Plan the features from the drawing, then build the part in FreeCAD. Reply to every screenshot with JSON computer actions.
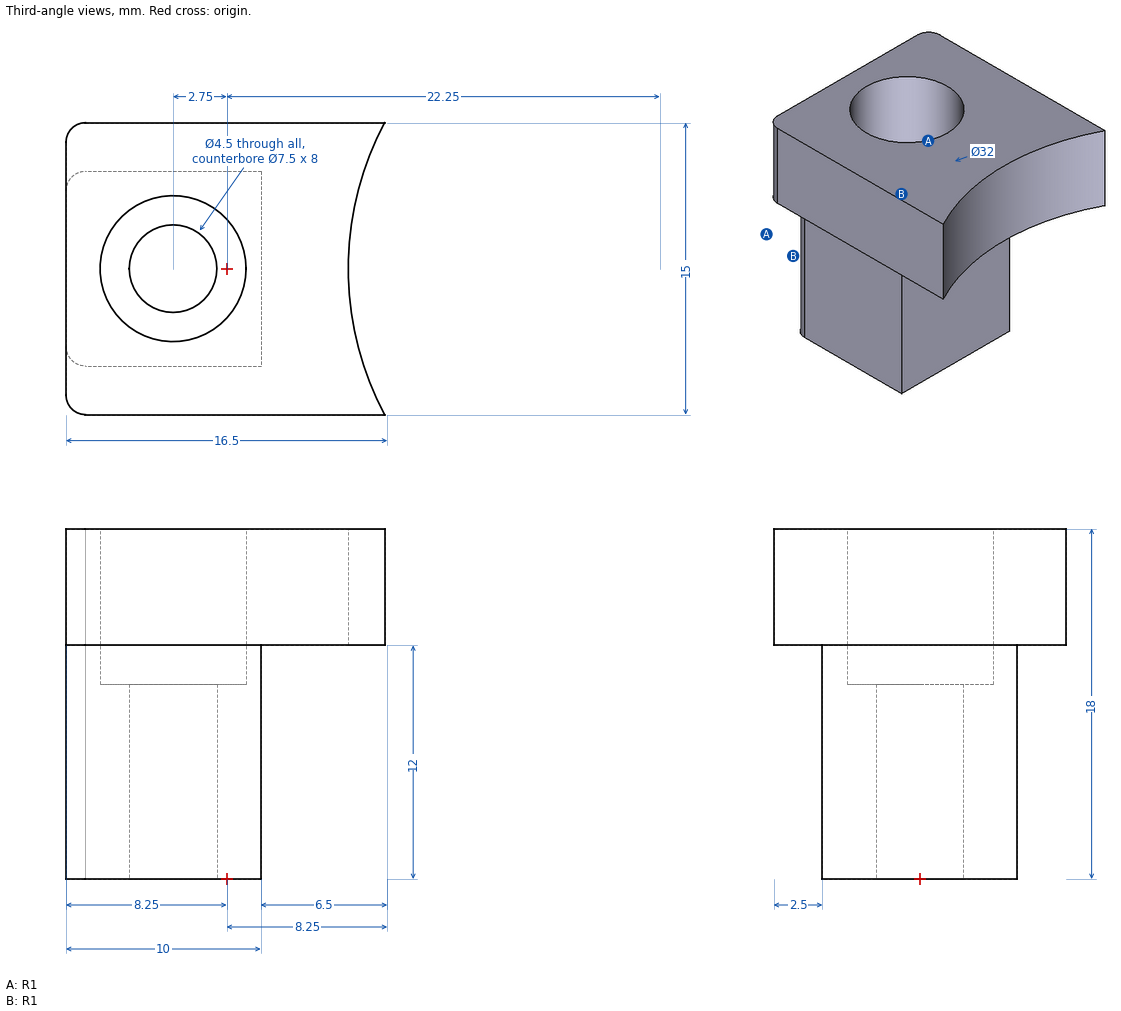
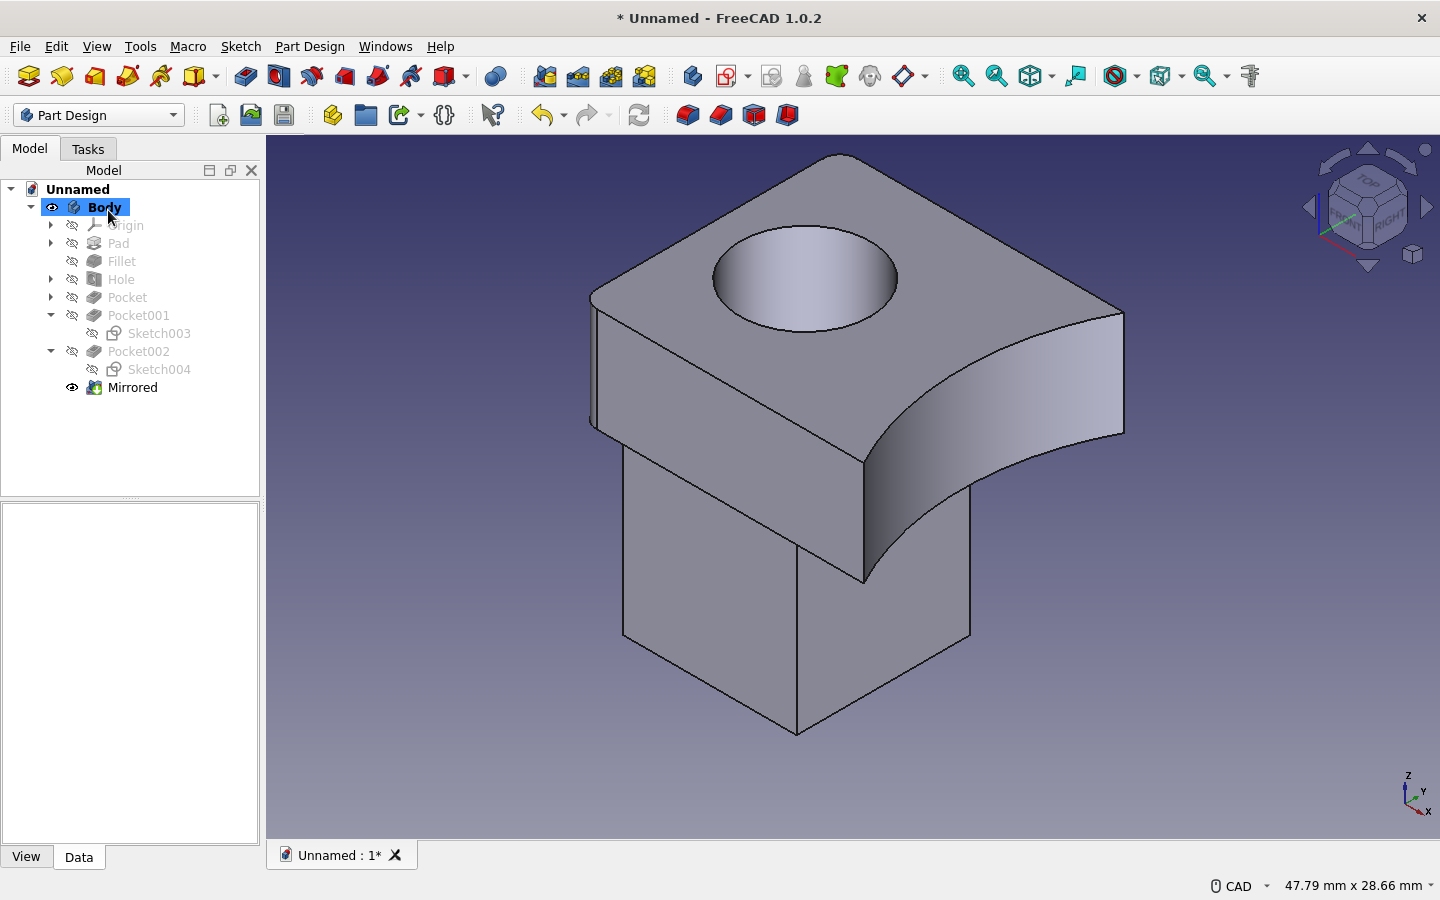
{"action": "key", "text": "1"}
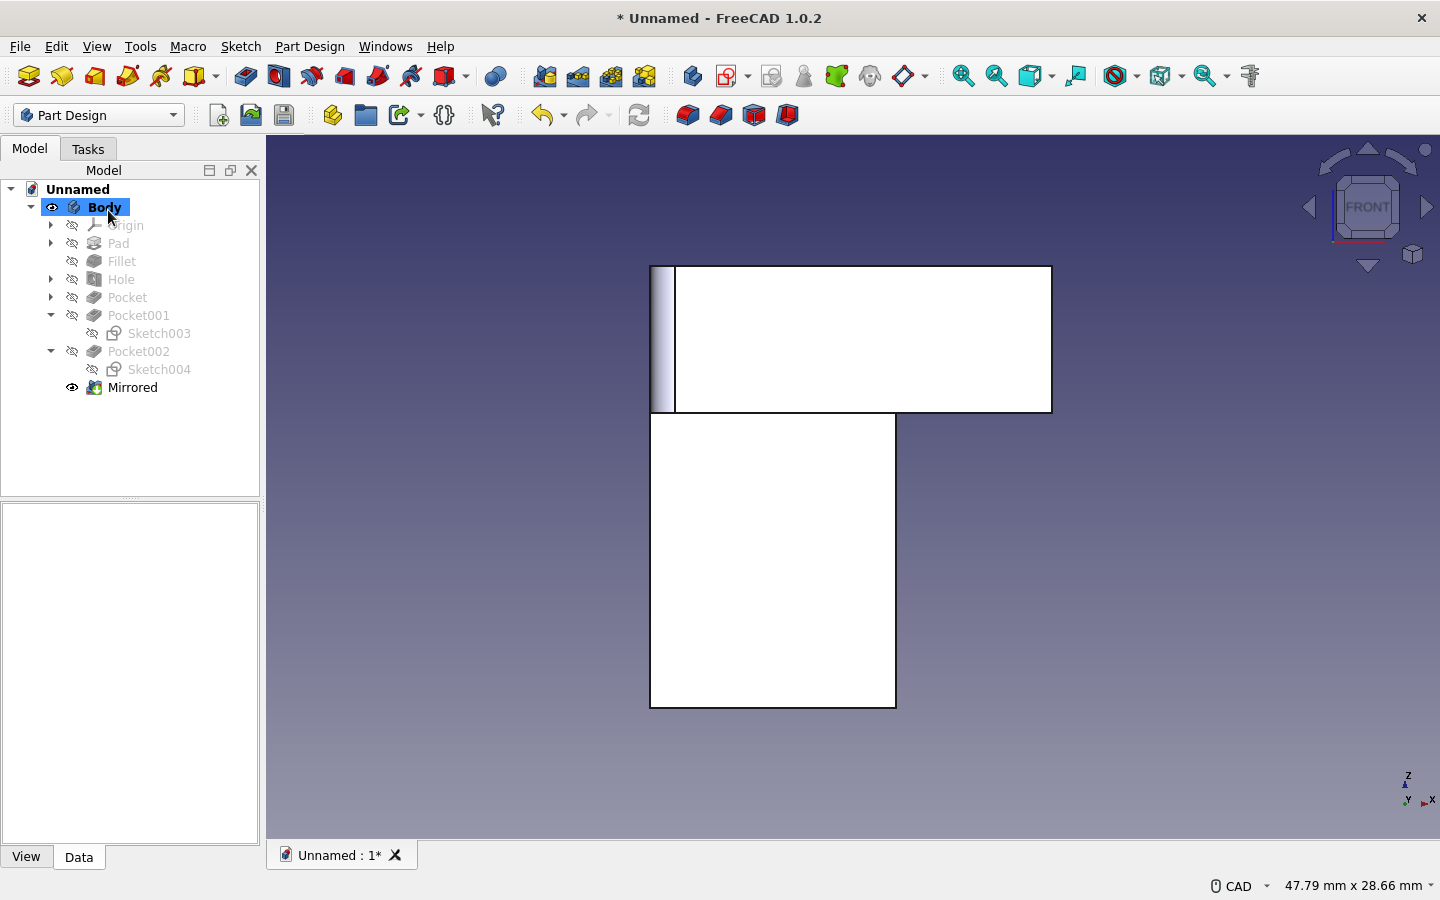
{"action": "left_click", "coordinate": [650, 560]}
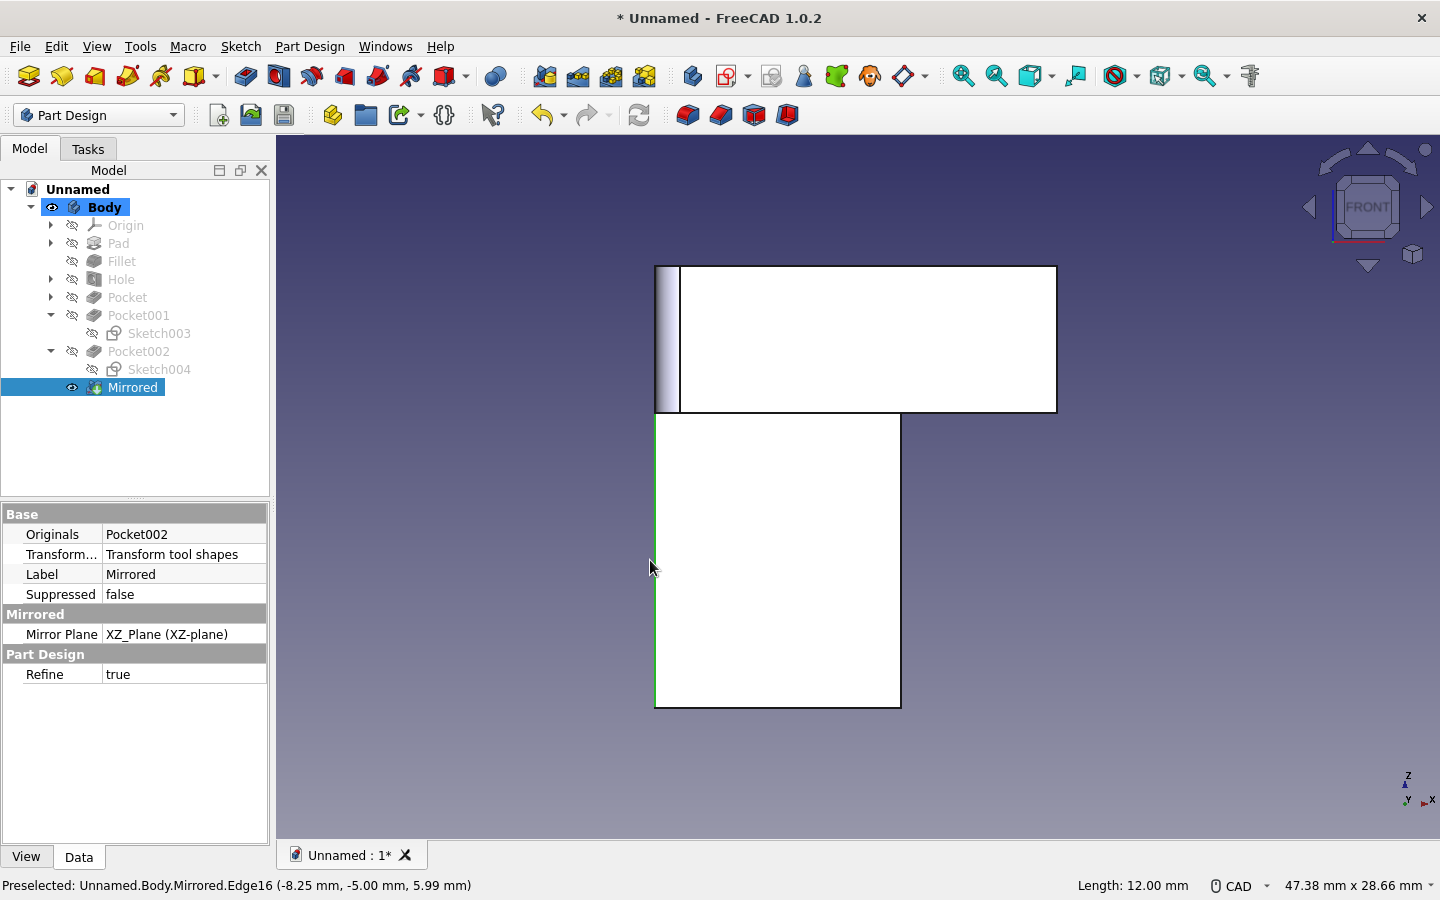
{"action": "key", "text": "3"}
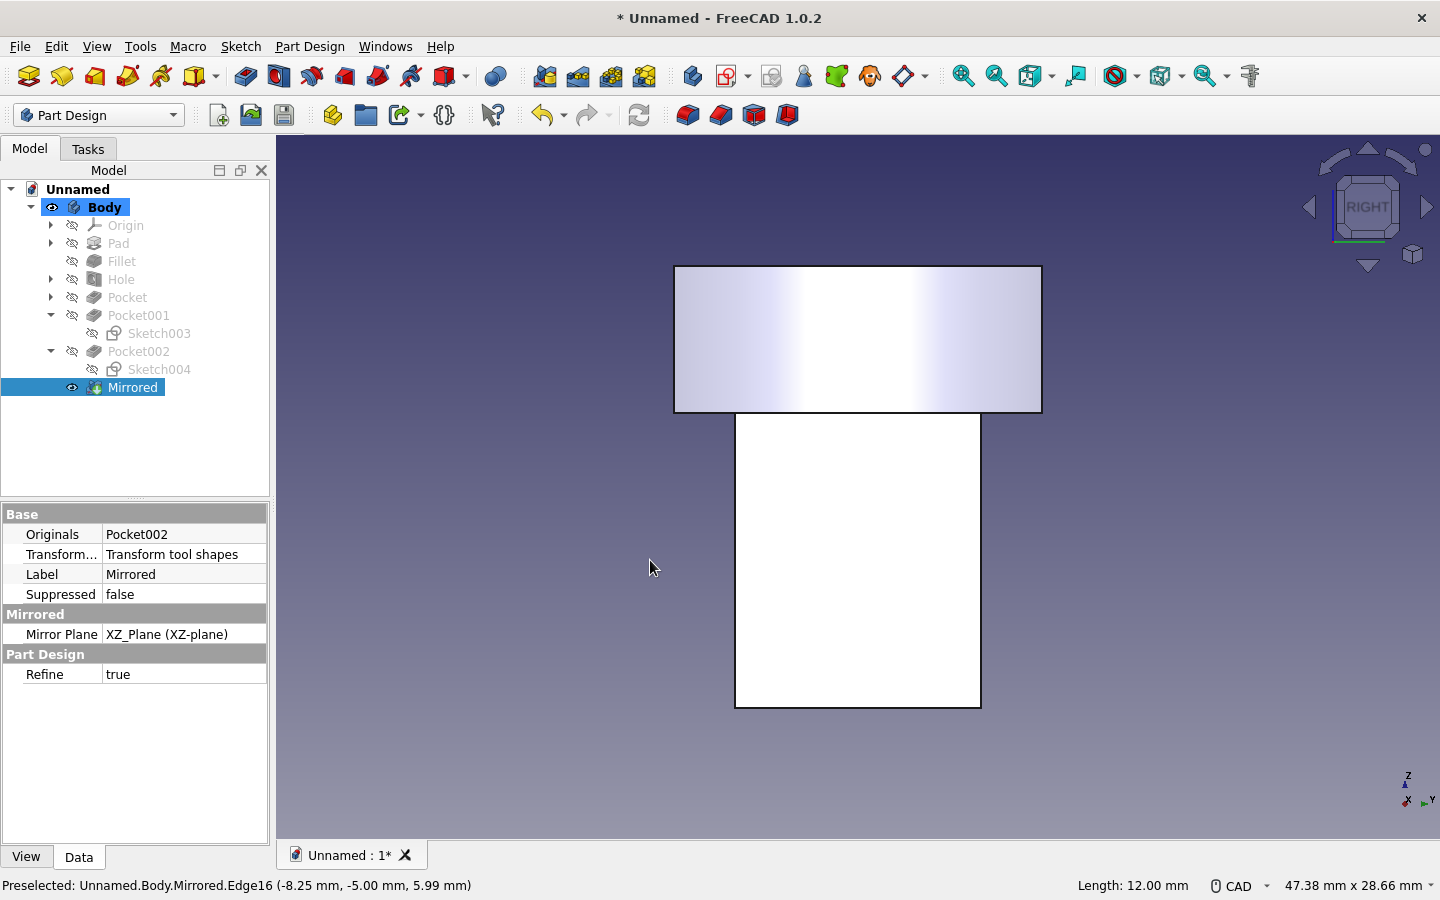
{"action": "key", "text": "5"}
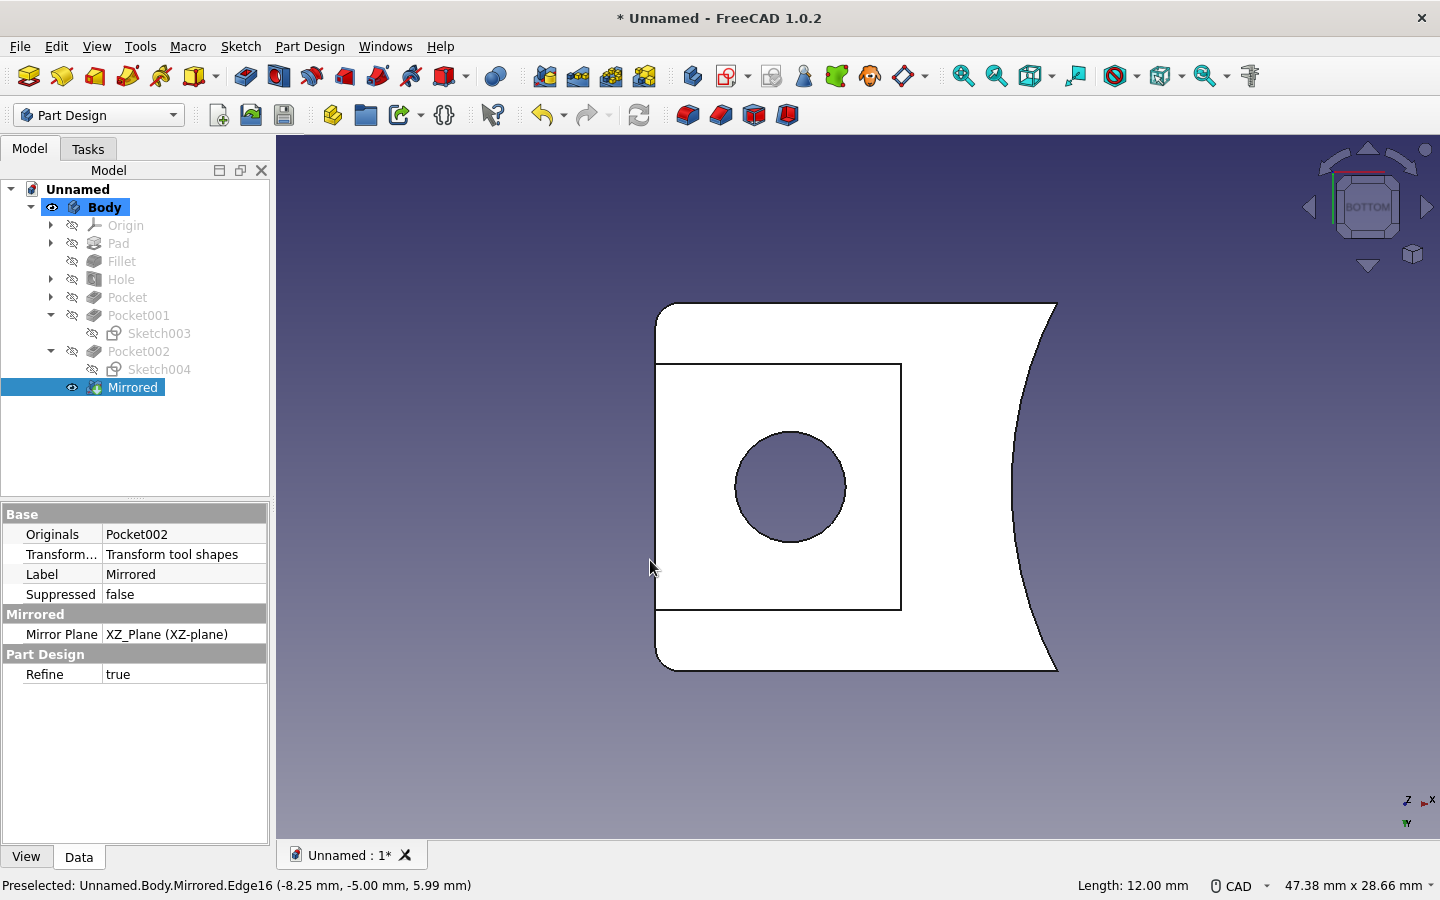
{"action": "key", "text": "4"}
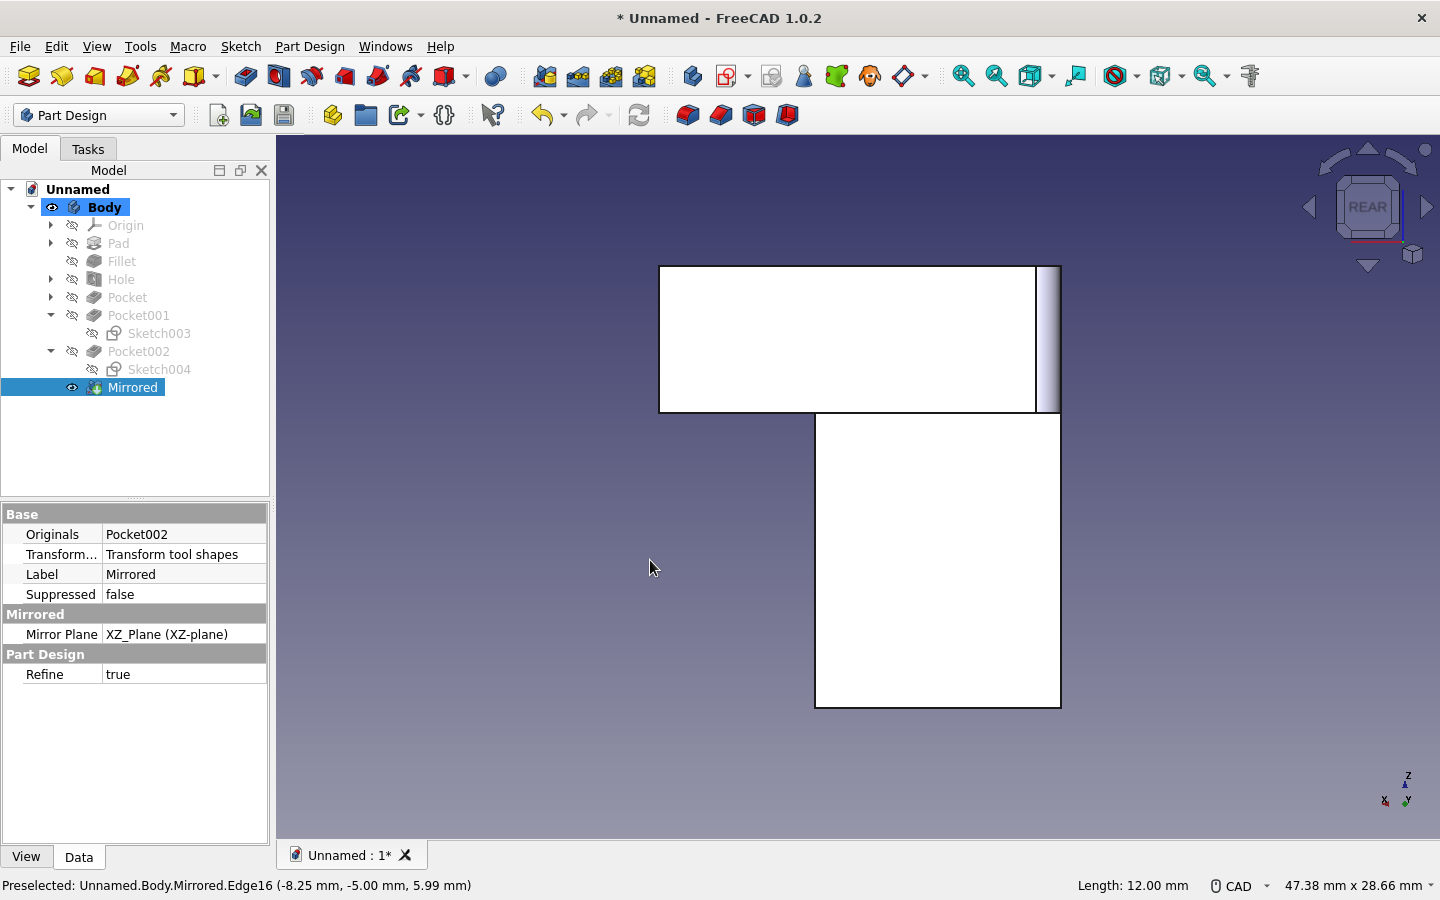
{"action": "left_click", "coordinate": [1061, 560], "text": "ctrl"}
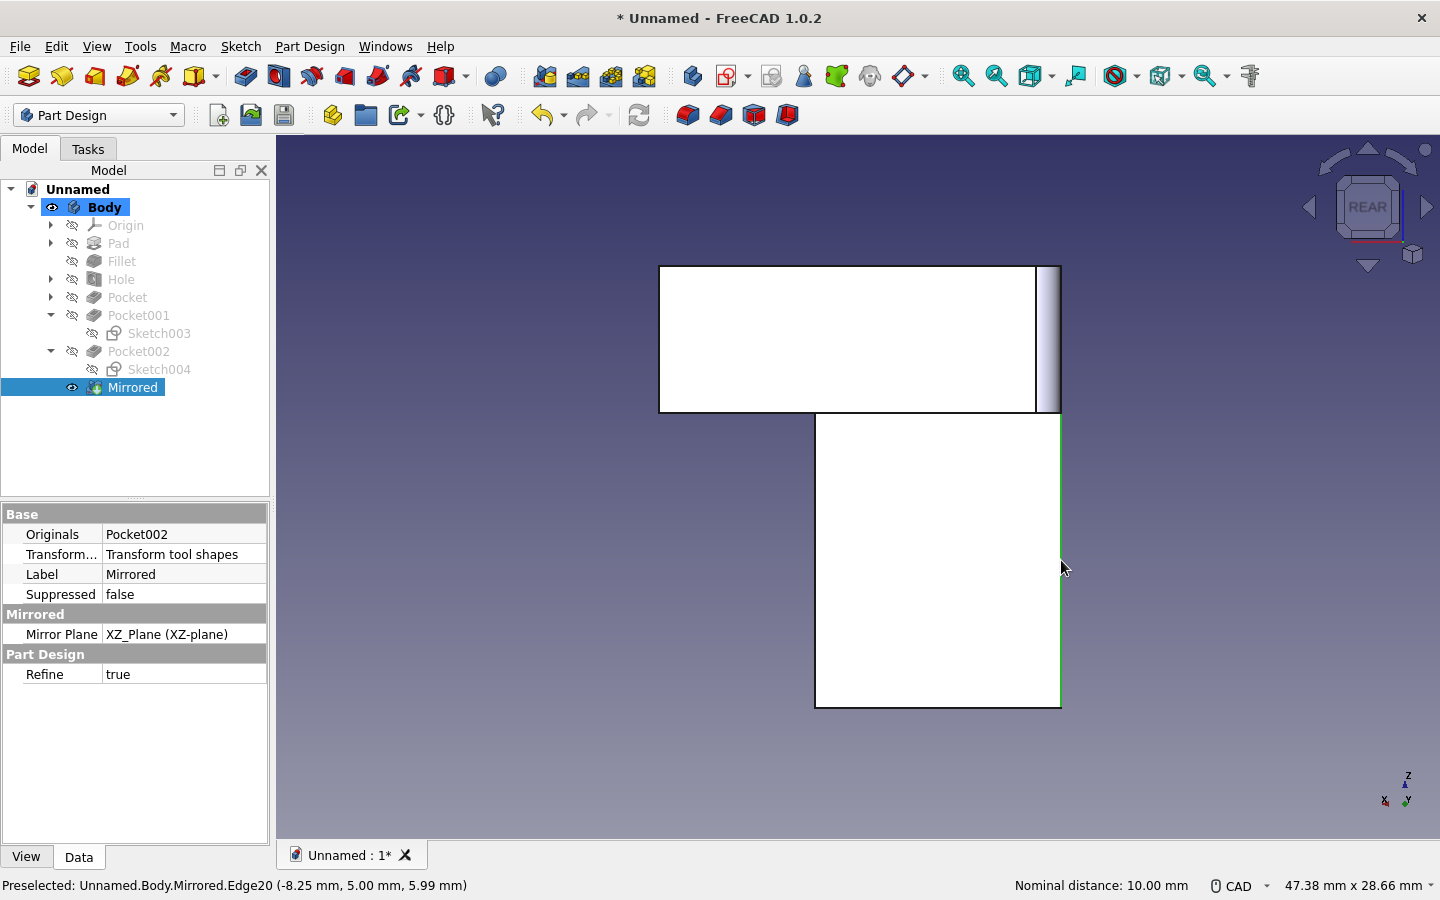
{"action": "left_click", "coordinate": [688, 116]}